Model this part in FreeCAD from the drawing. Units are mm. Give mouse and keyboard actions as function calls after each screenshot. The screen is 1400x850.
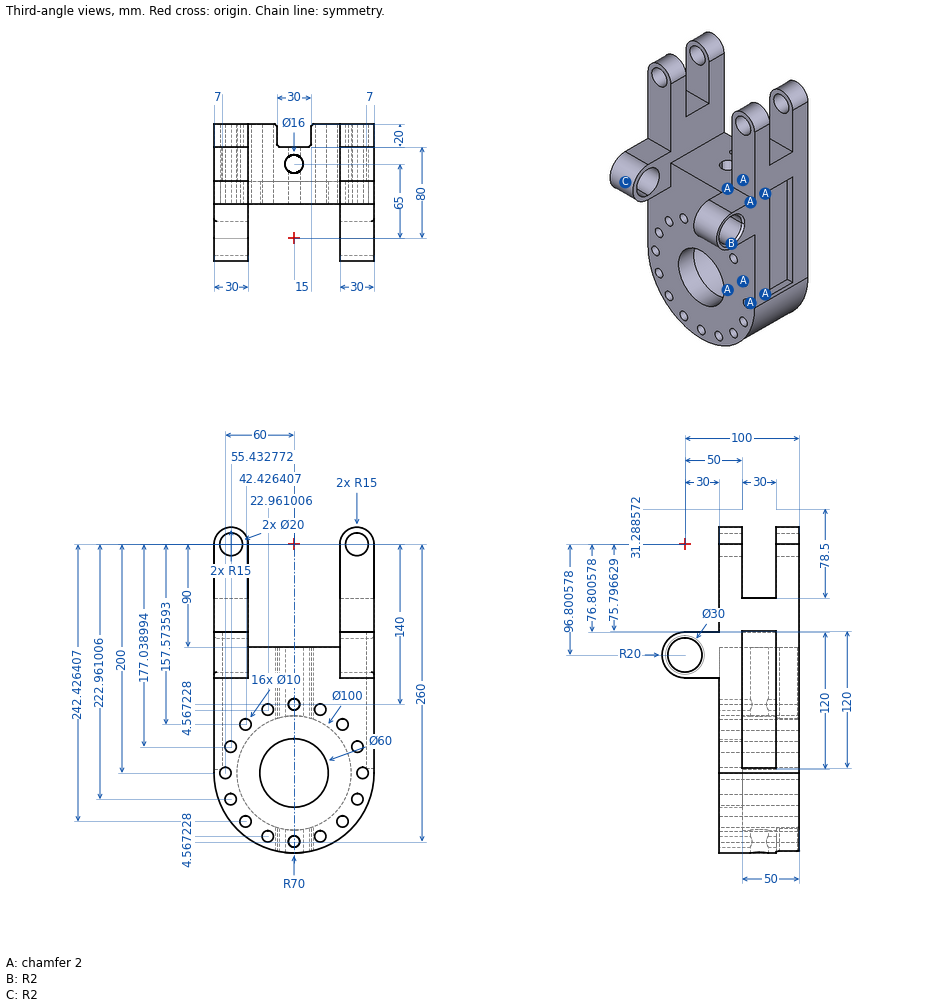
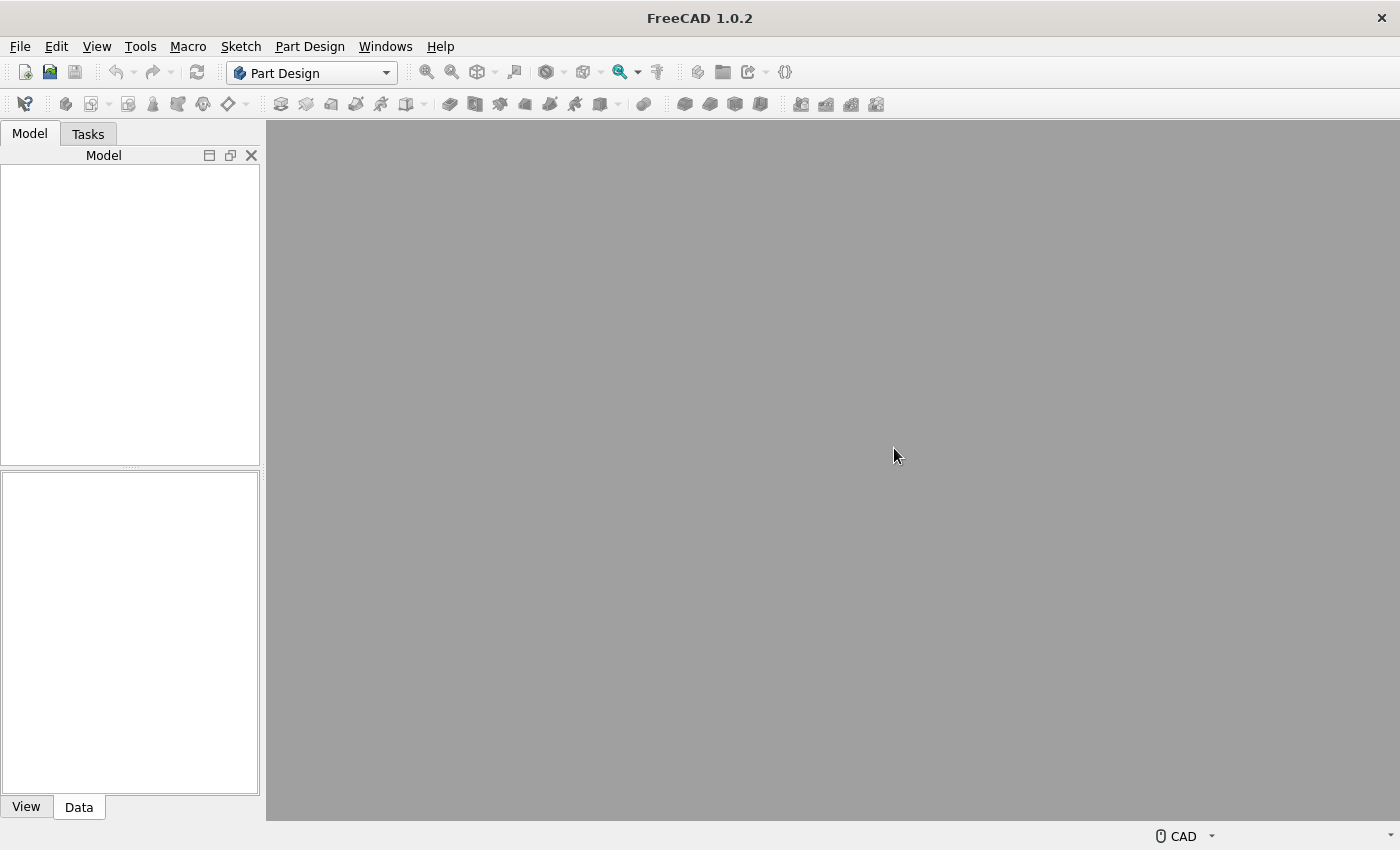
key(ctrl+n)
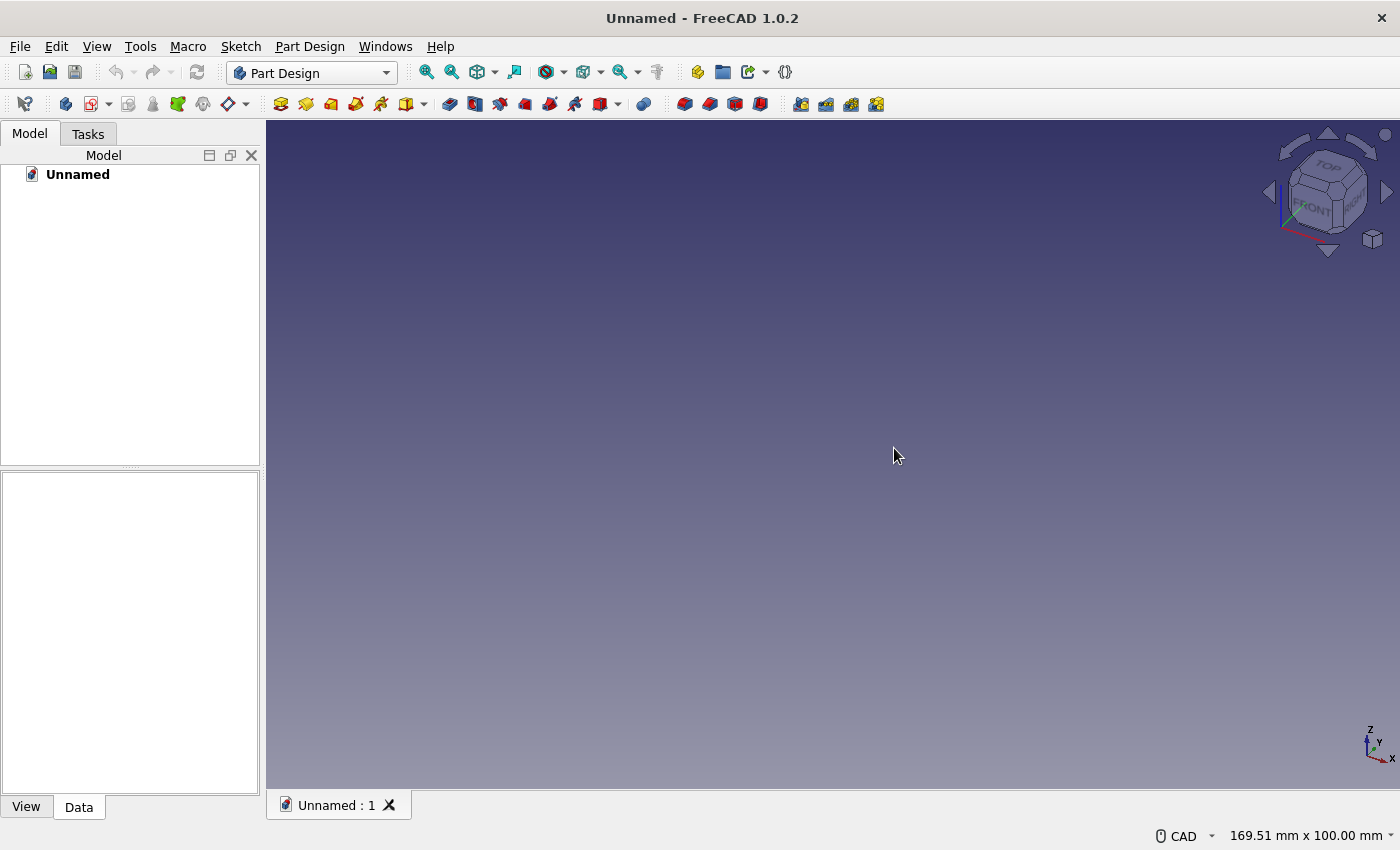
click(90, 104)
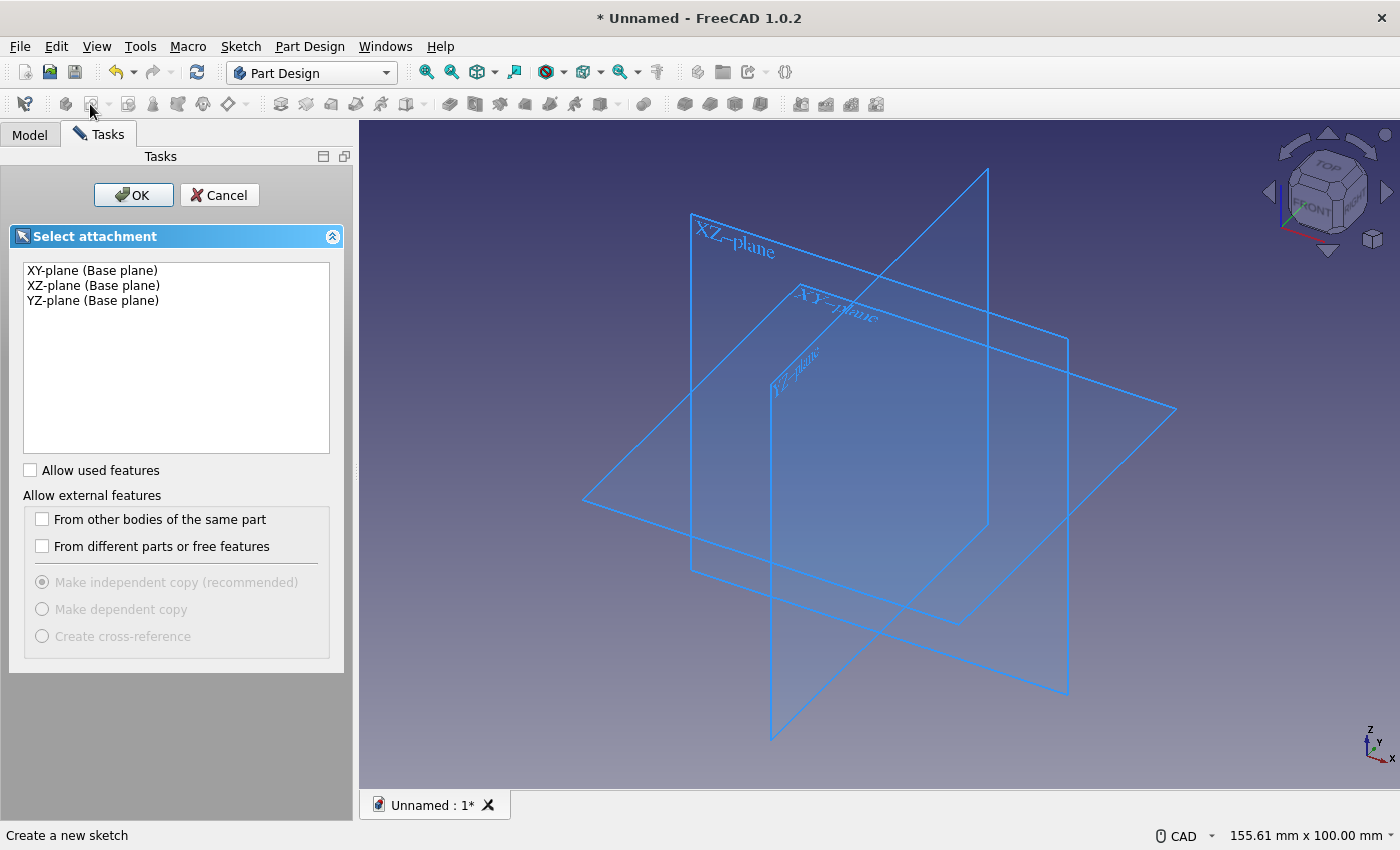
click(84, 286)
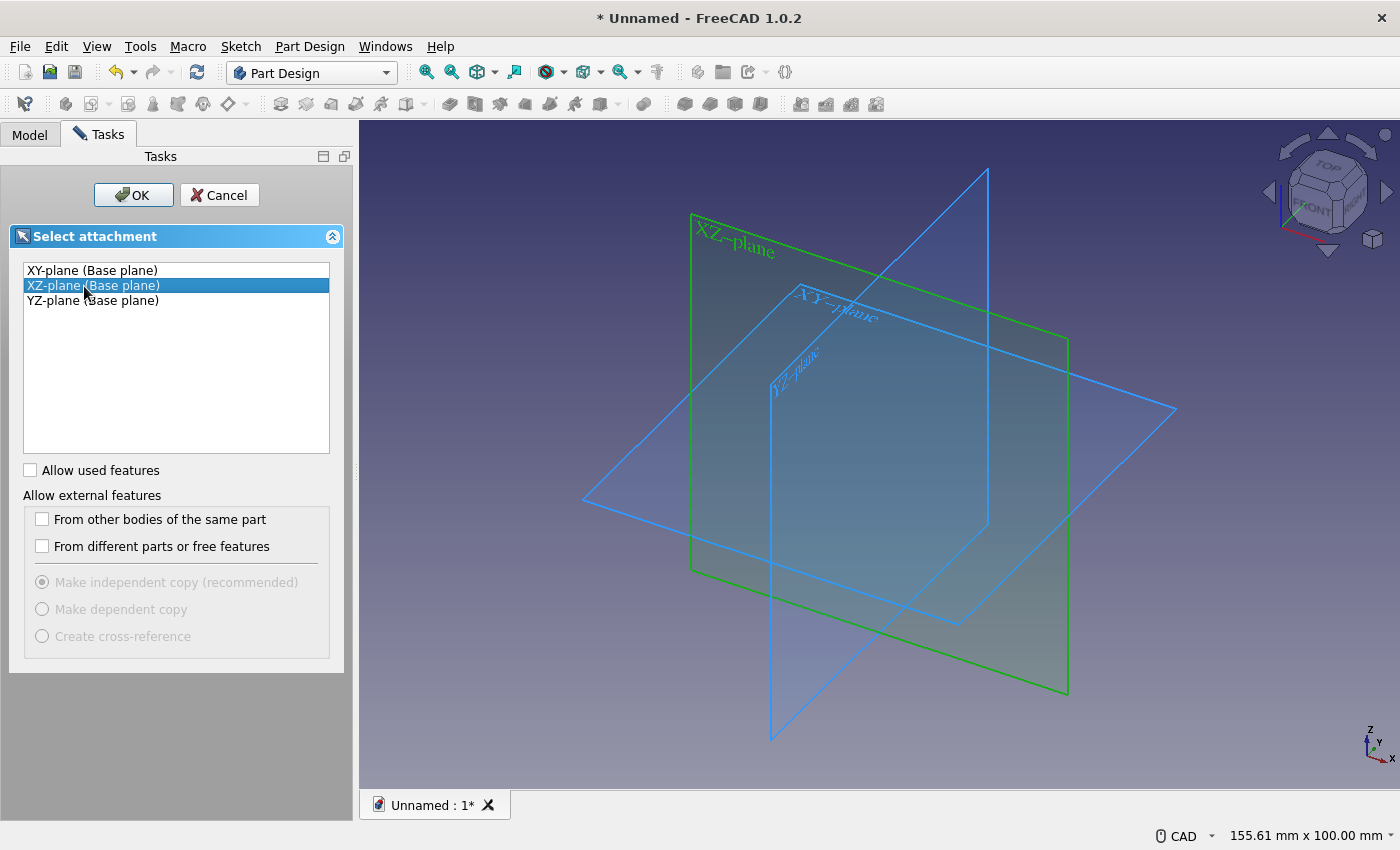
click(134, 195)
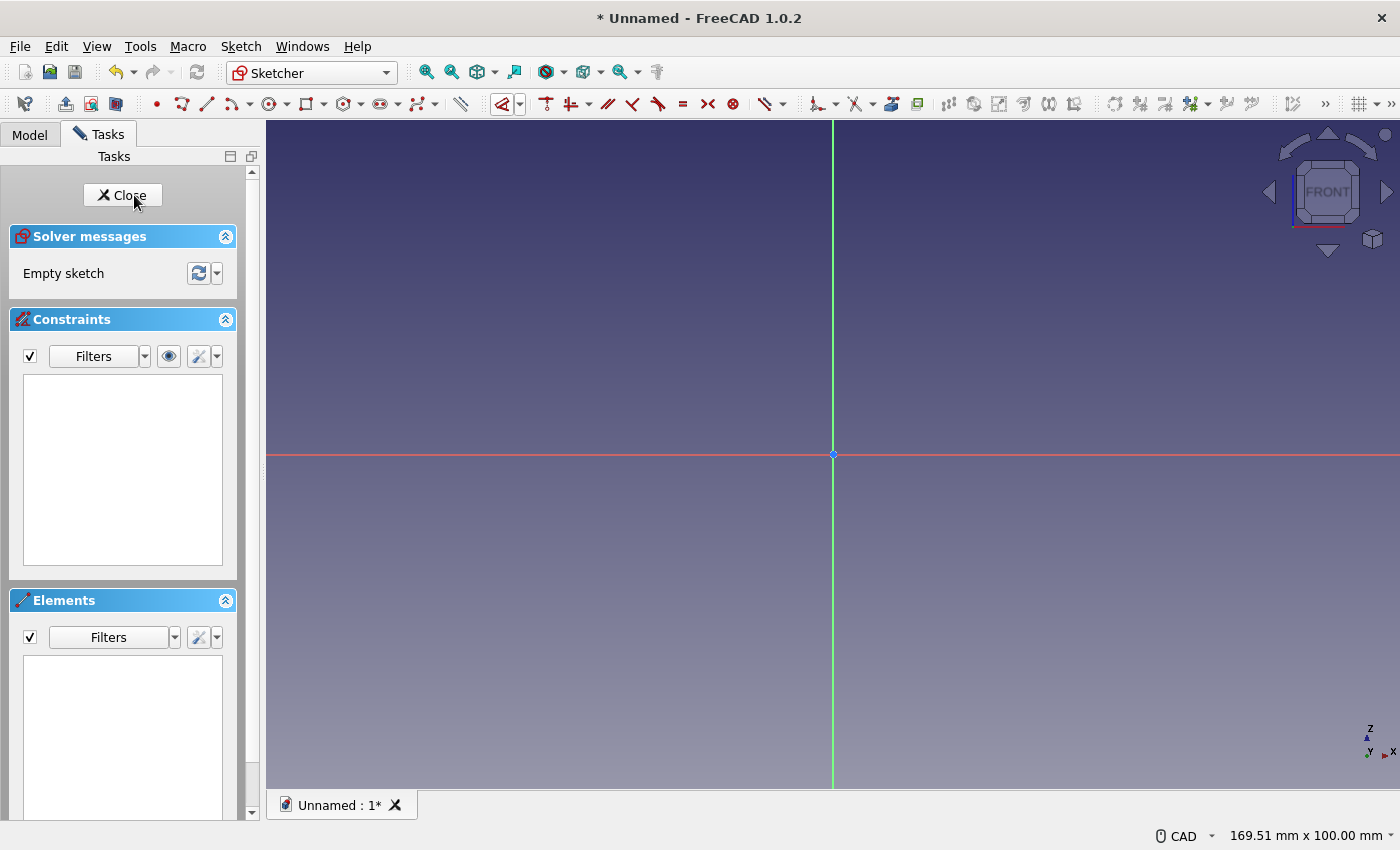
scroll(742, 175, down, 7)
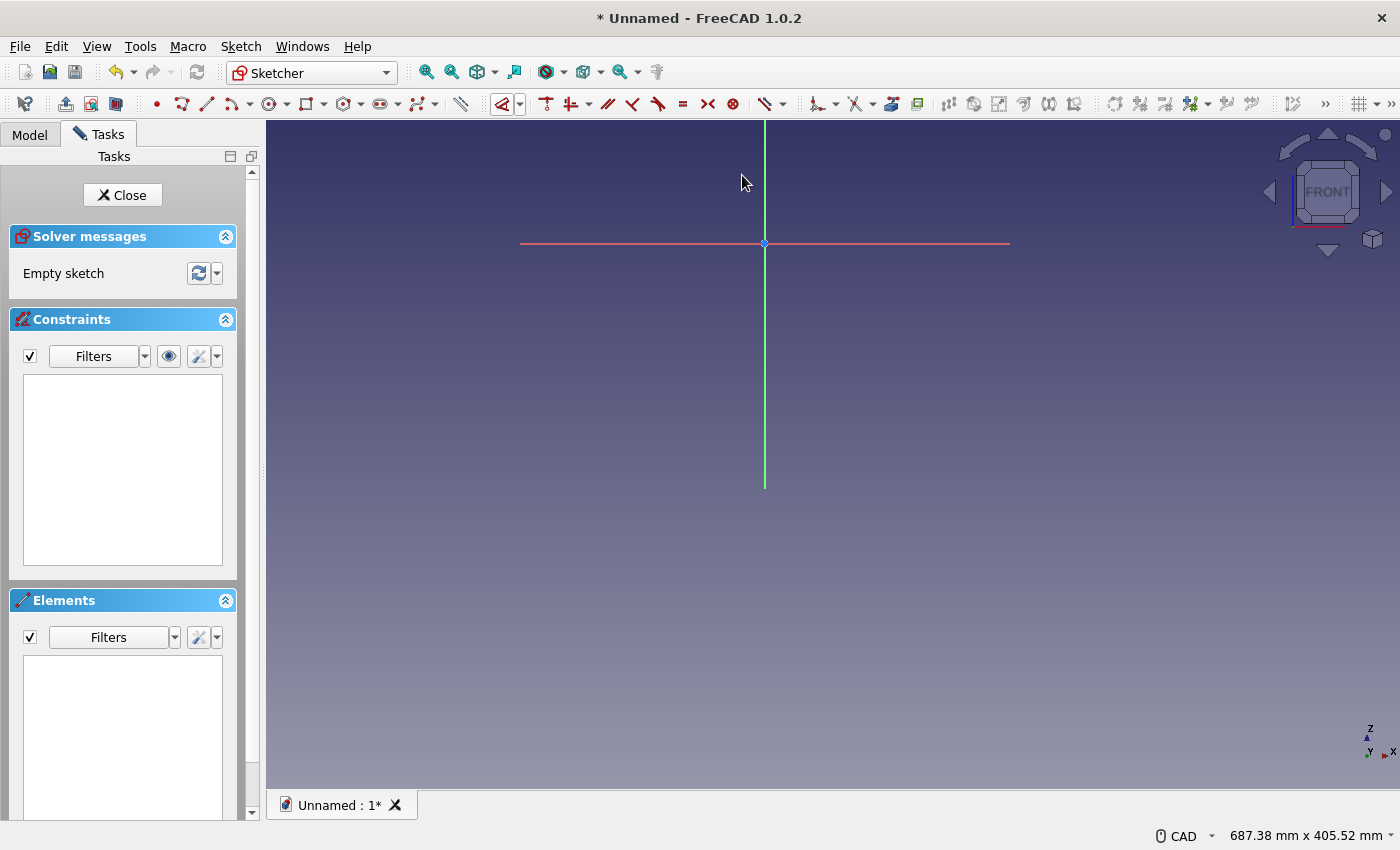
key(g)
key(l)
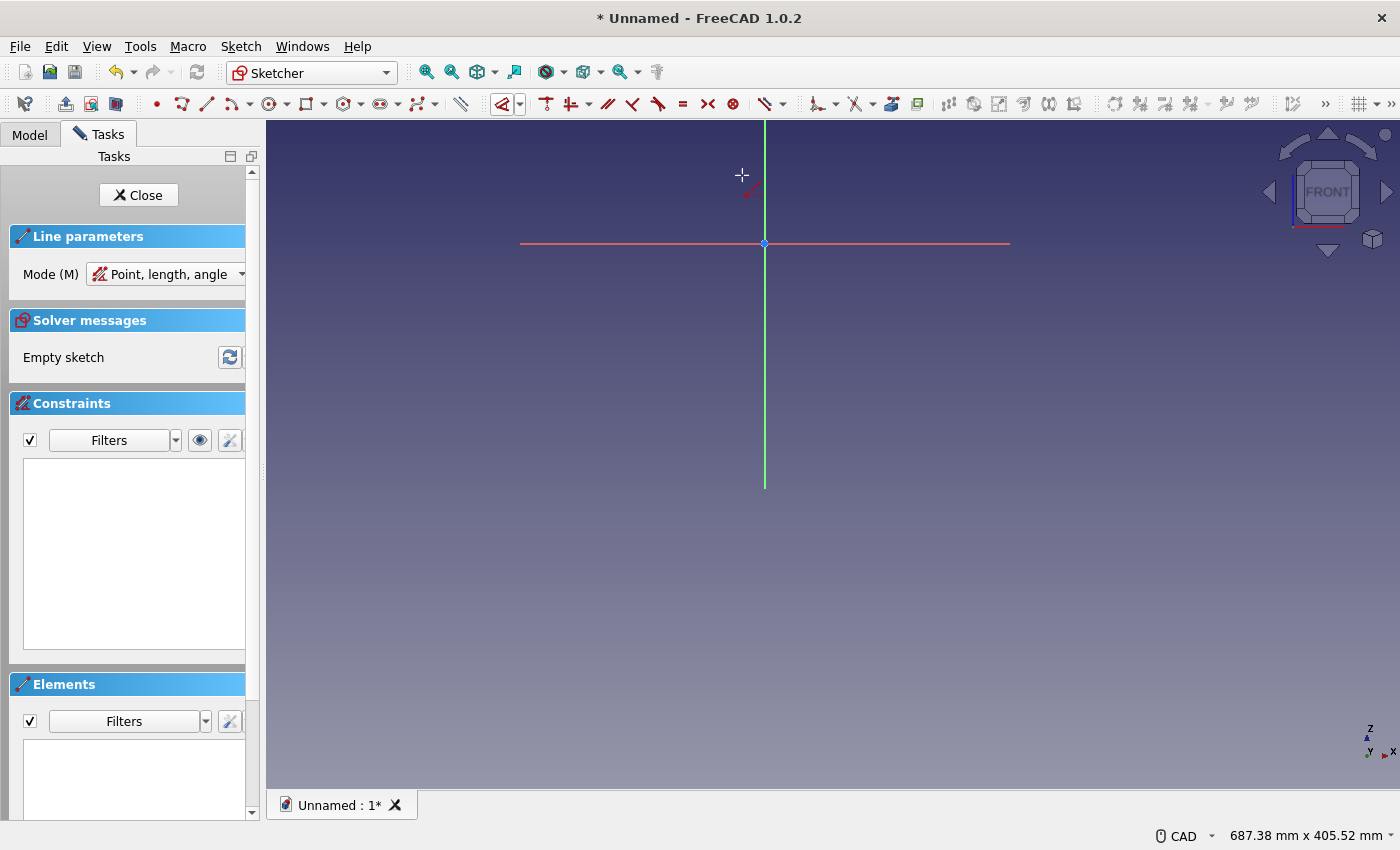
click(649, 574)
click(649, 244)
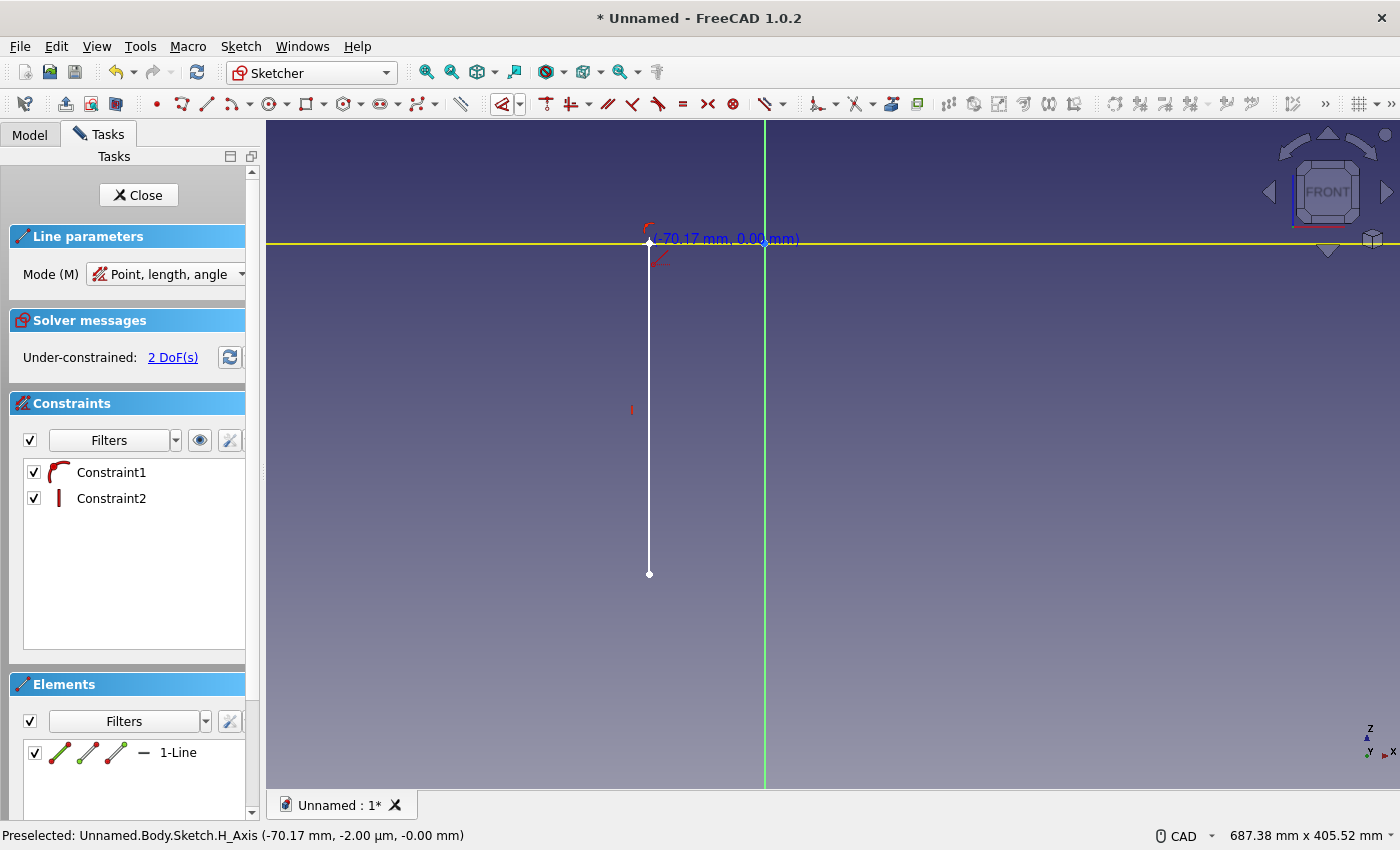
key(g)
key(m)